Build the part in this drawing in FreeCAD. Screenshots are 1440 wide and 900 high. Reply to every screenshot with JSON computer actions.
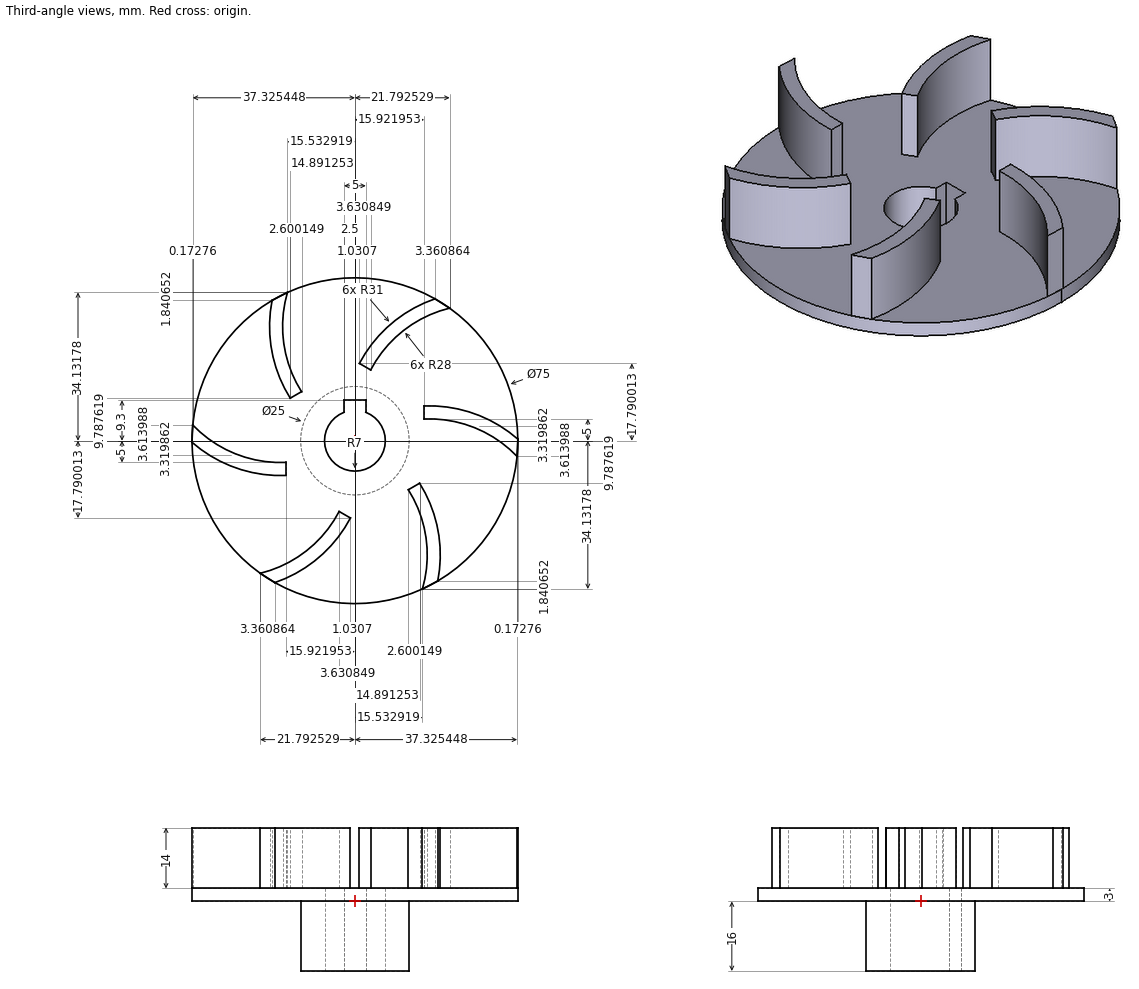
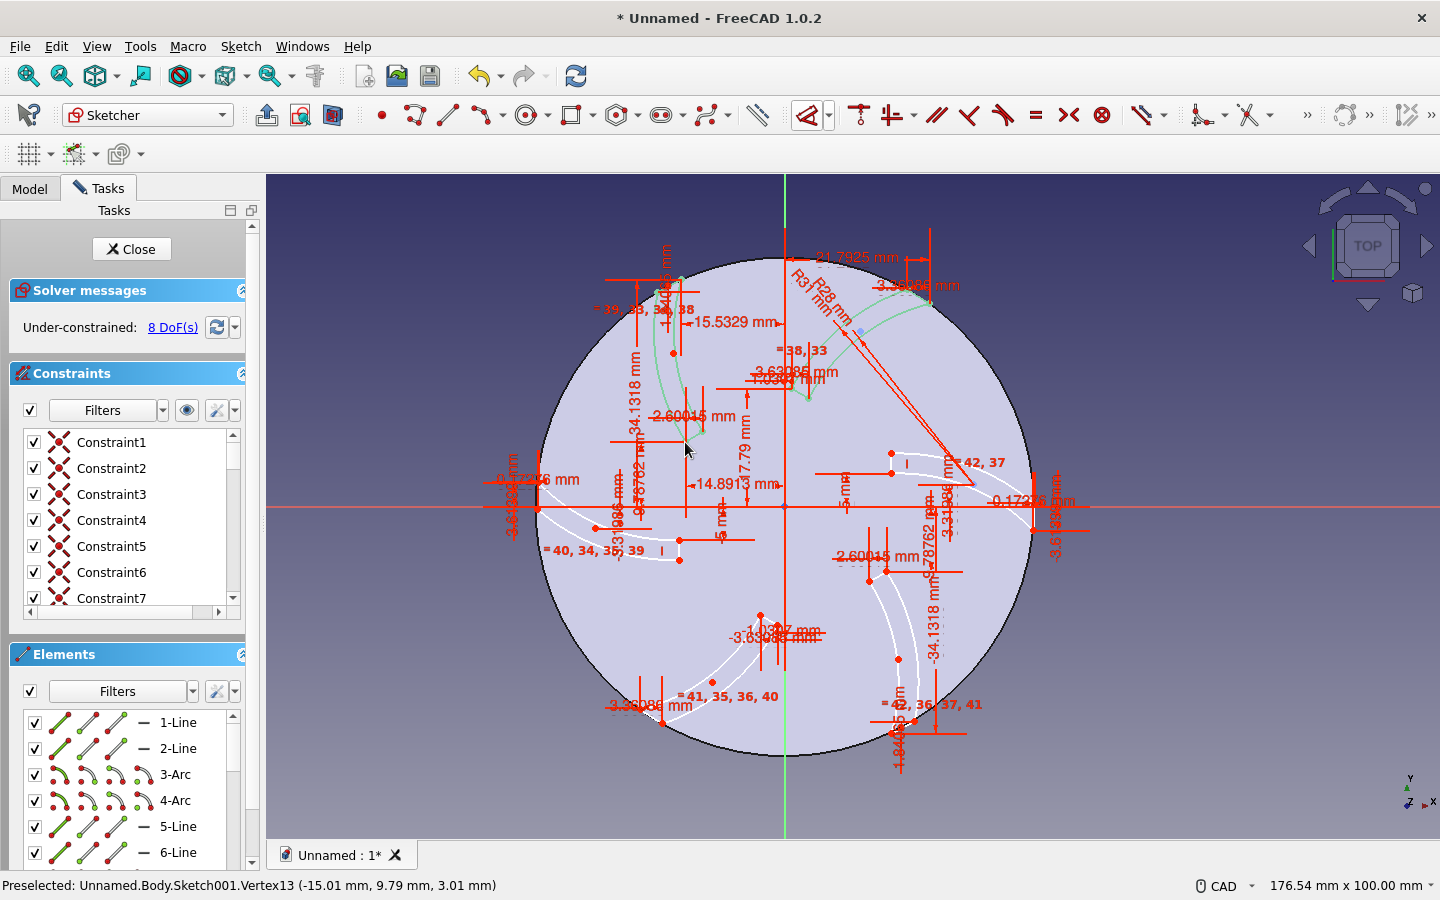
{"action": "left_click", "coordinate": [539, 483]}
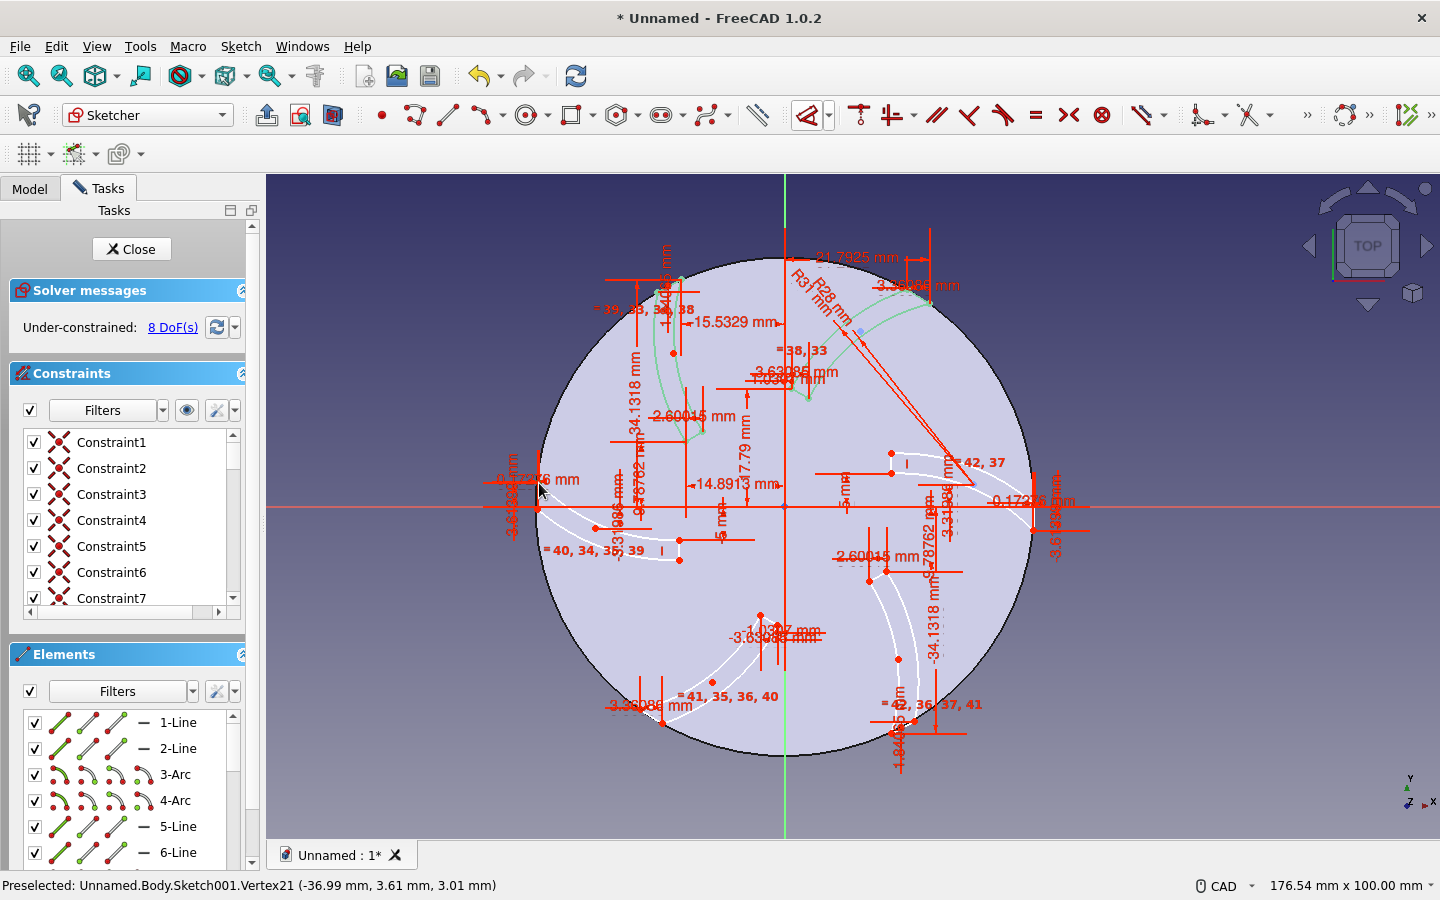
{"action": "left_click", "coordinate": [828, 116]}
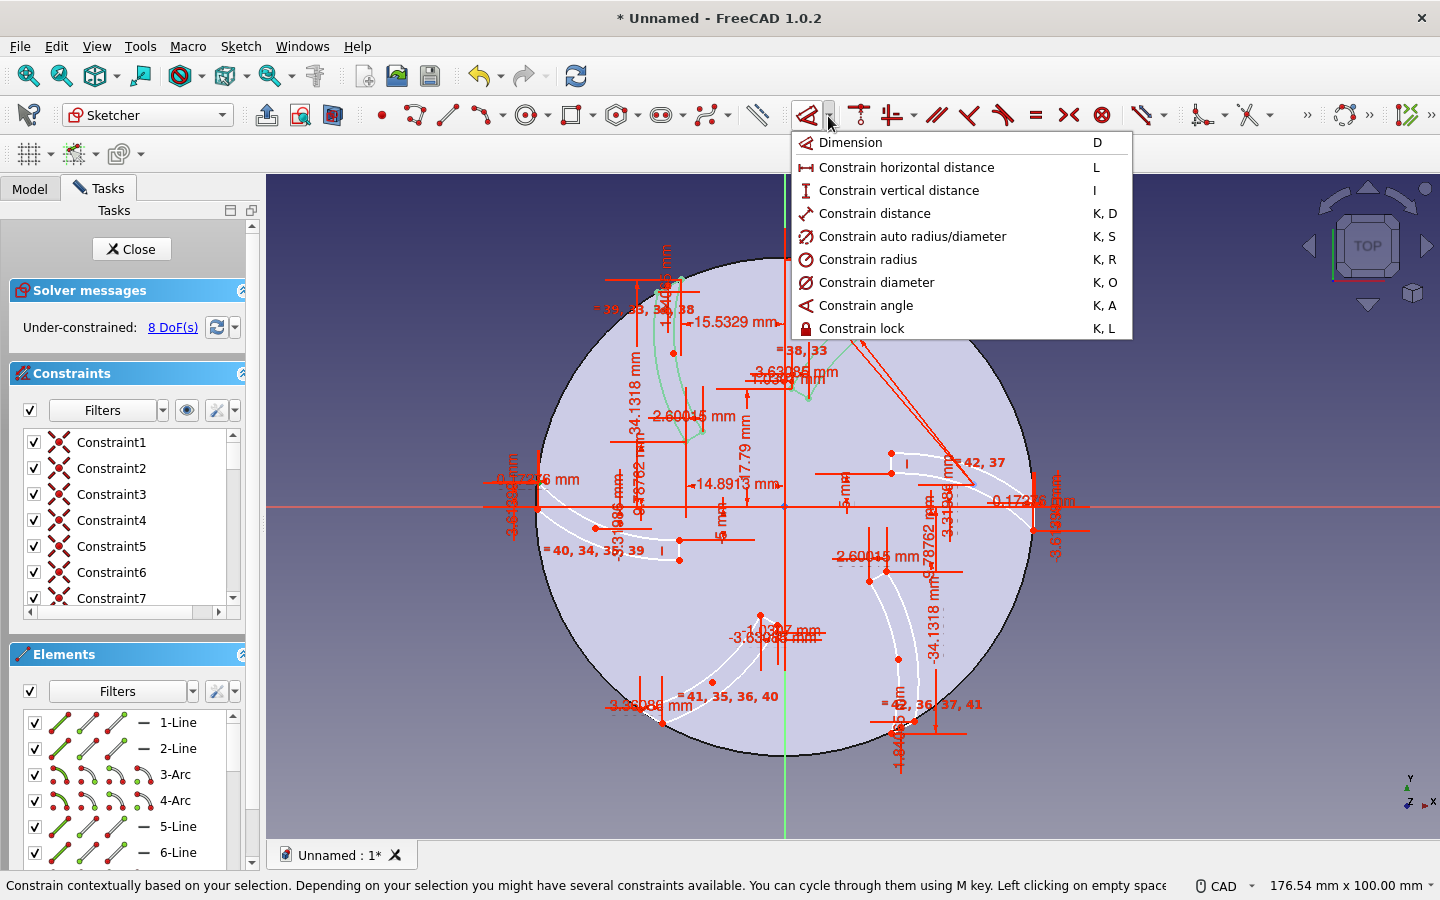
{"action": "left_click", "coordinate": [962, 168]}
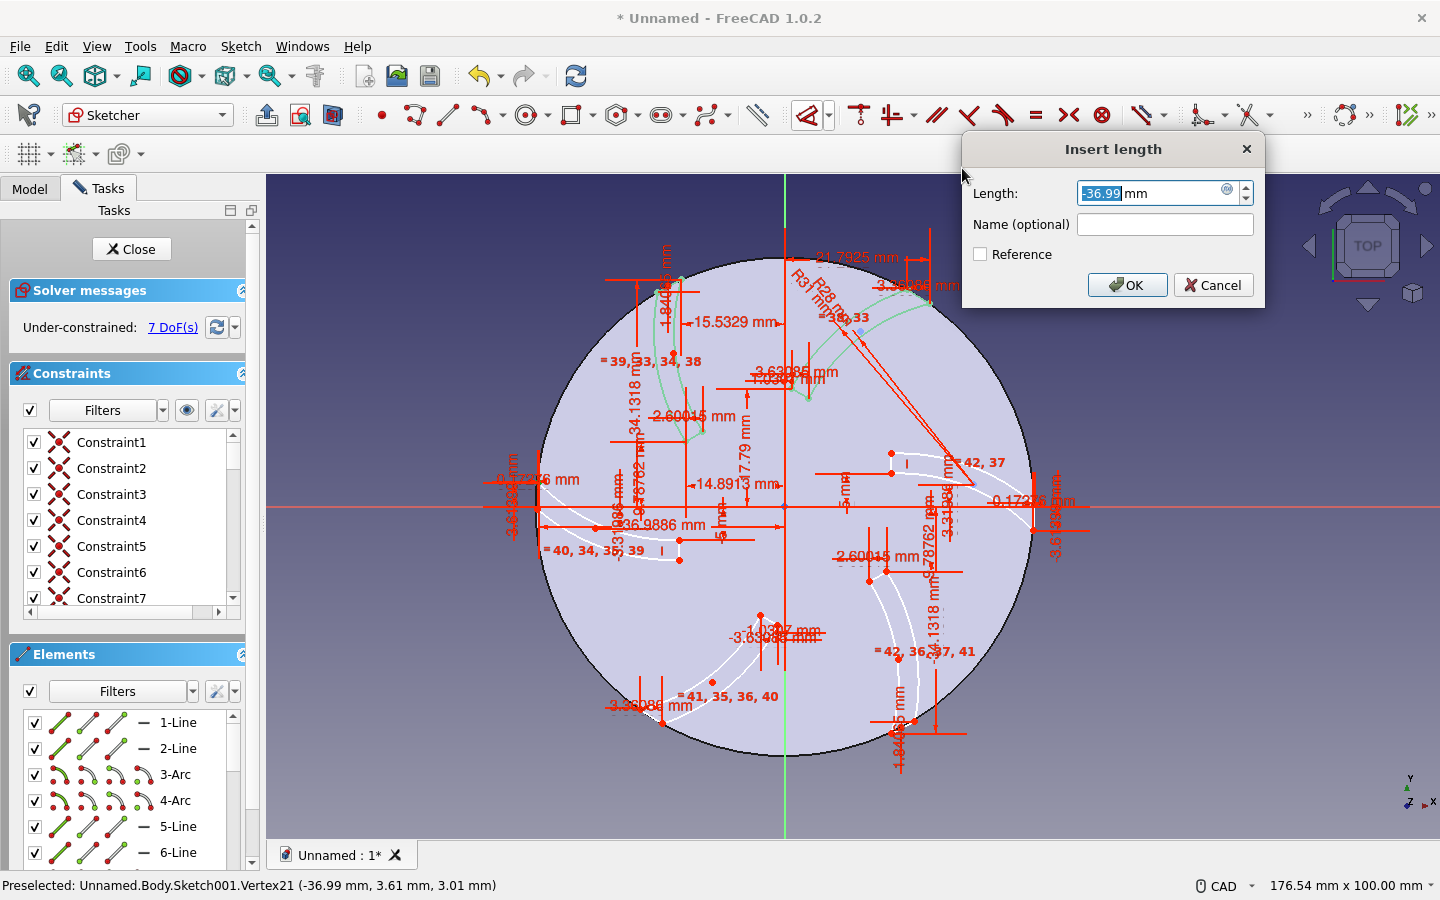
{"action": "type", "text": "-37.325448"}
{"action": "key", "text": "Return"}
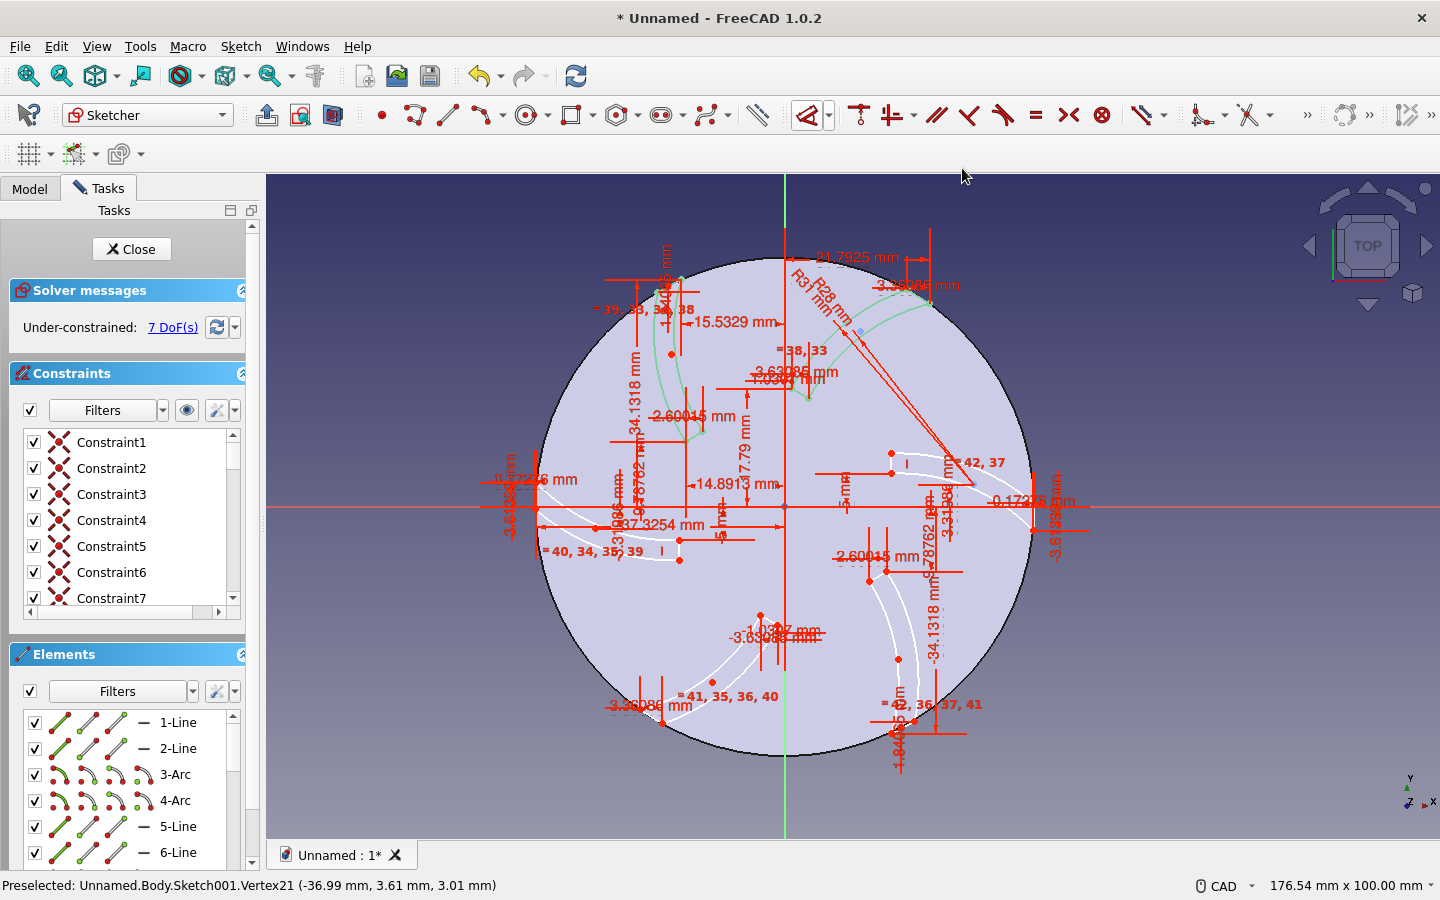
{"action": "left_click", "coordinate": [679, 560]}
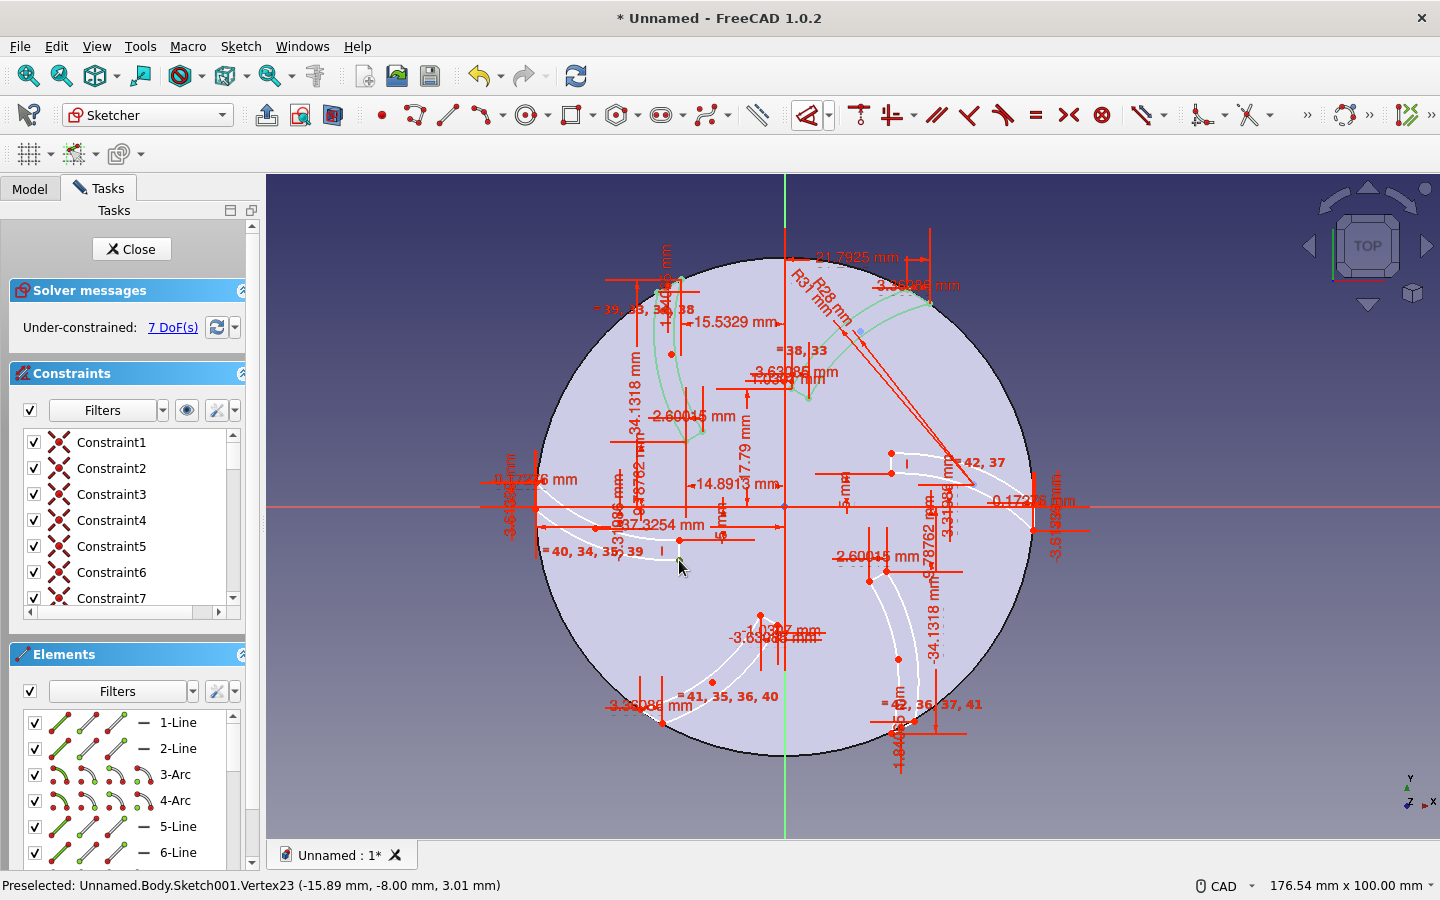
{"action": "key", "text": "l"}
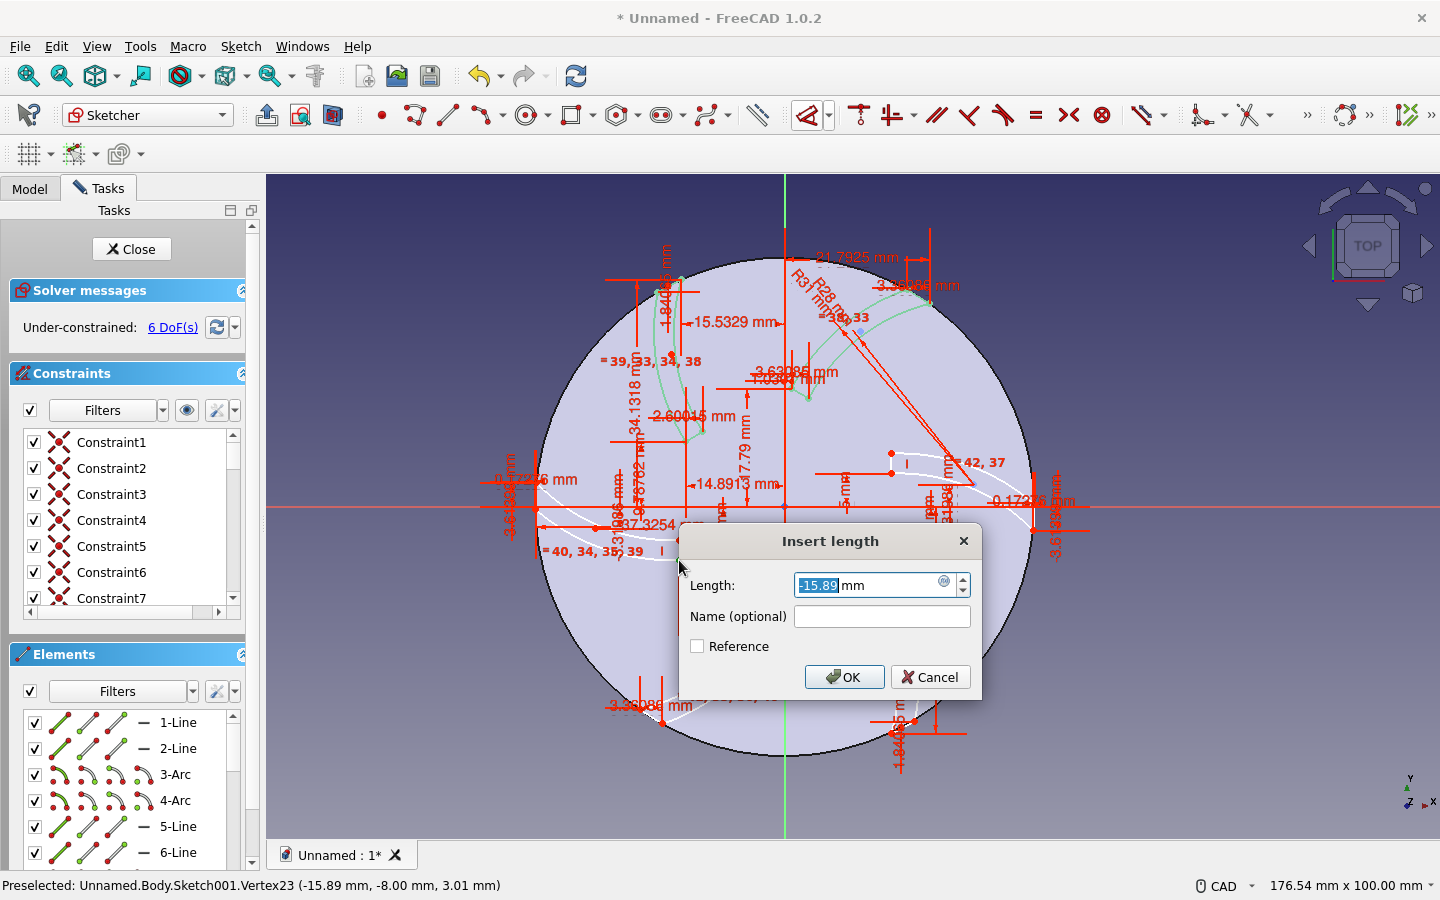
{"action": "type", "text": "-15.921953"}
{"action": "key", "text": "Return"}